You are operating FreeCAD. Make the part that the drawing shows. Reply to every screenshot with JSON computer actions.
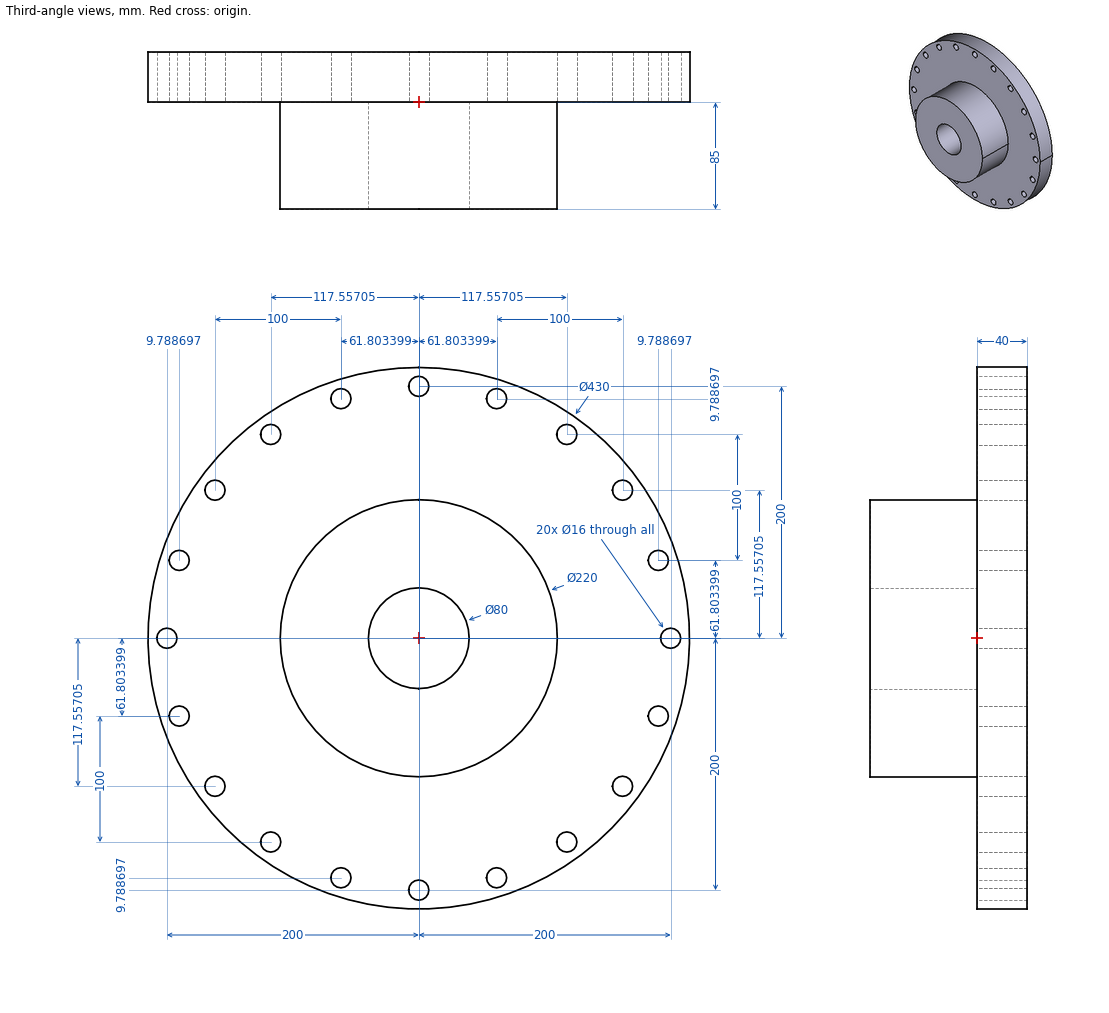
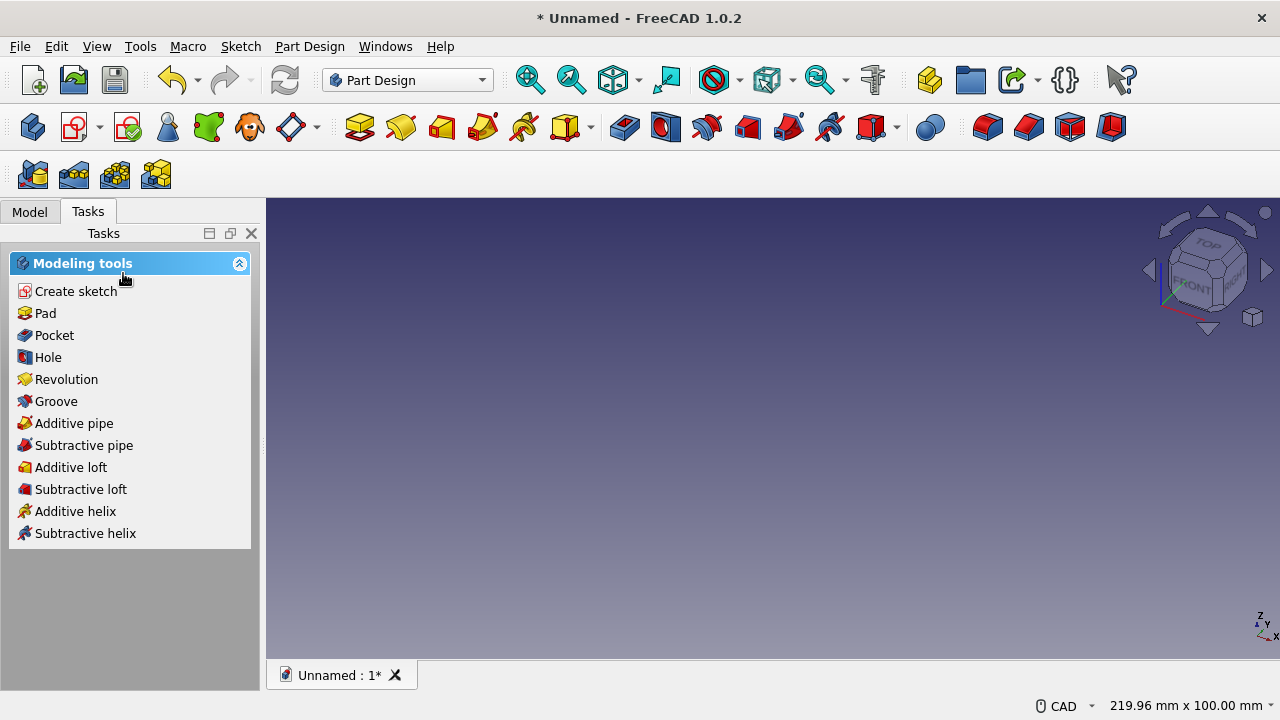
{"action": "left_click", "coordinate": [360, 128]}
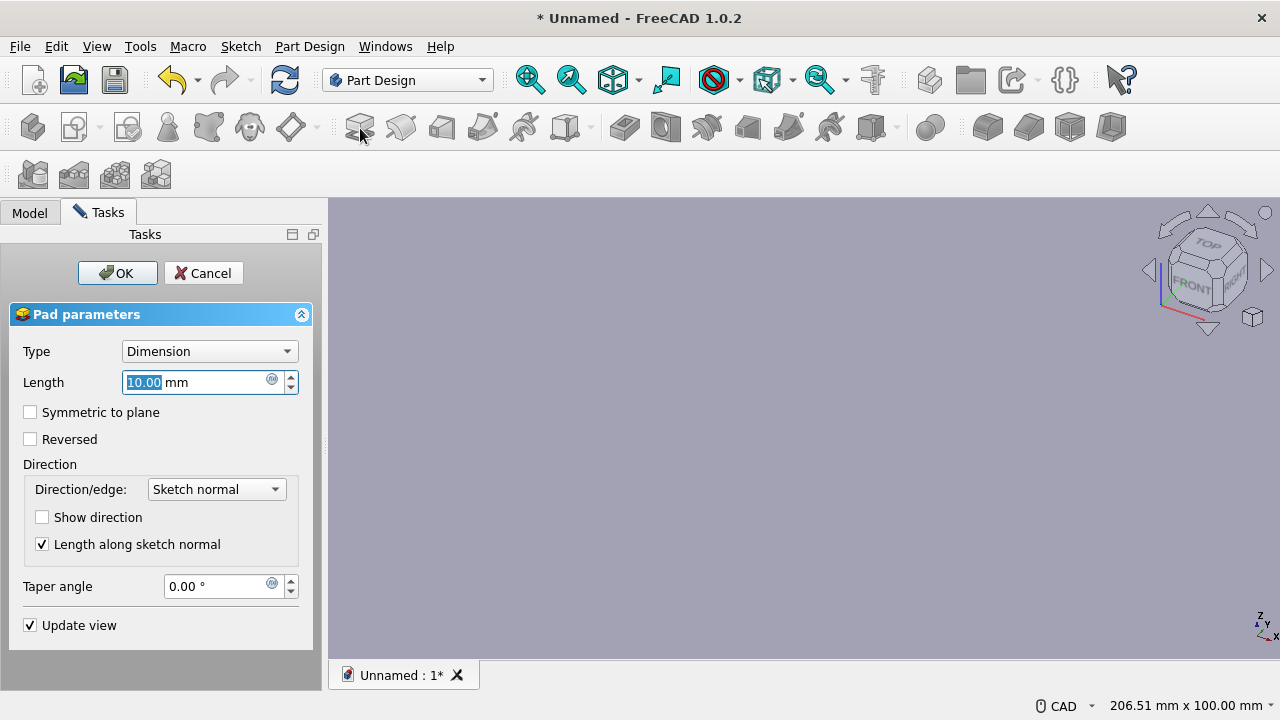
{"action": "type", "text": "40"}
{"action": "key", "text": "Tab"}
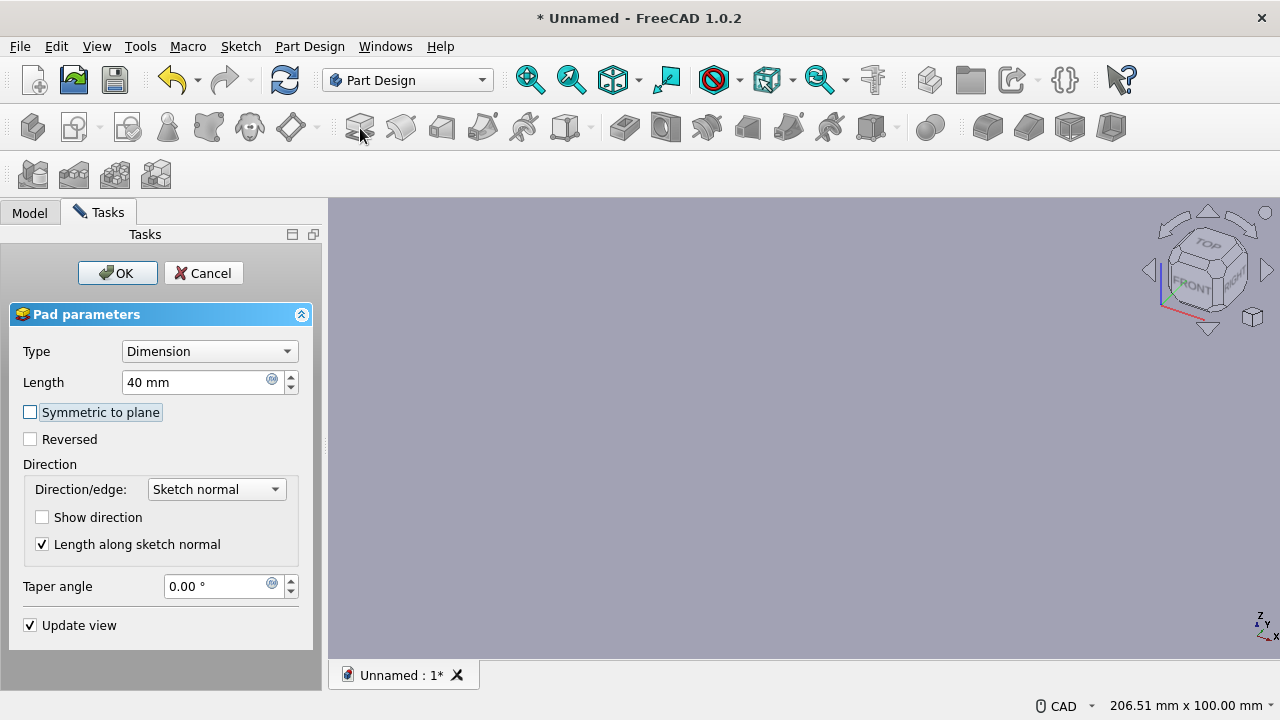
{"action": "left_click", "coordinate": [31, 439]}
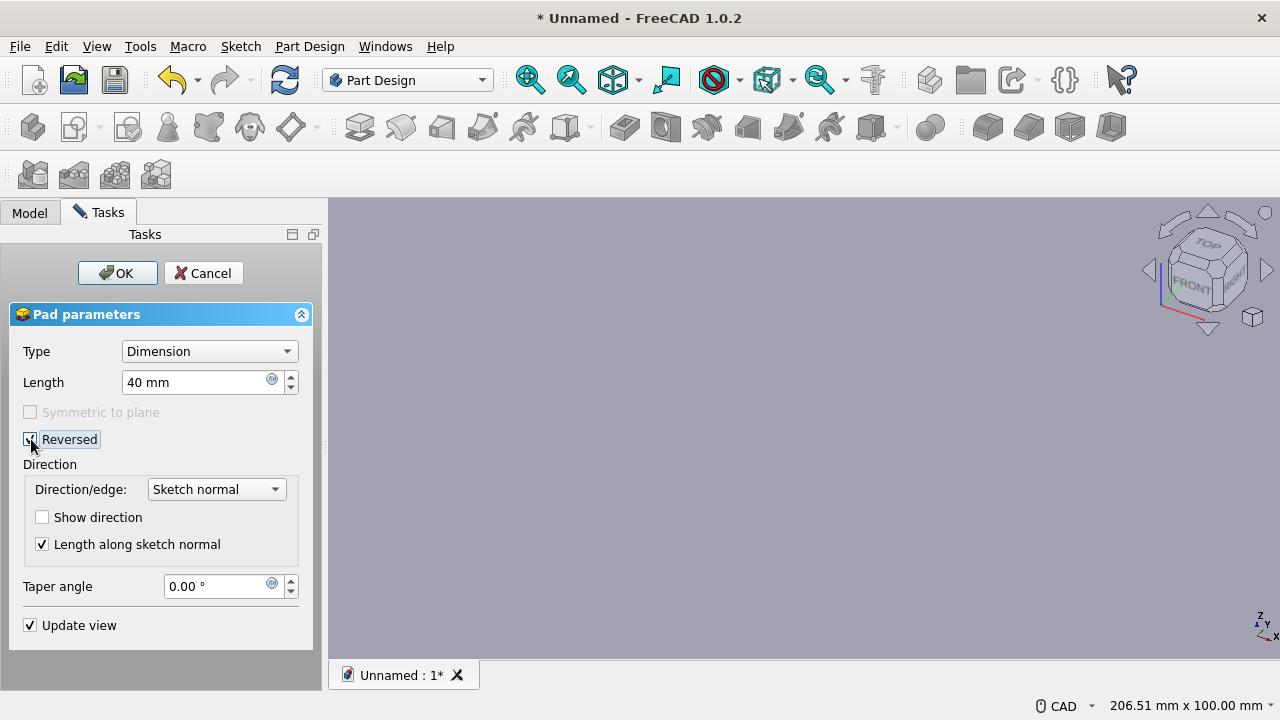
{"action": "left_click", "coordinate": [118, 273]}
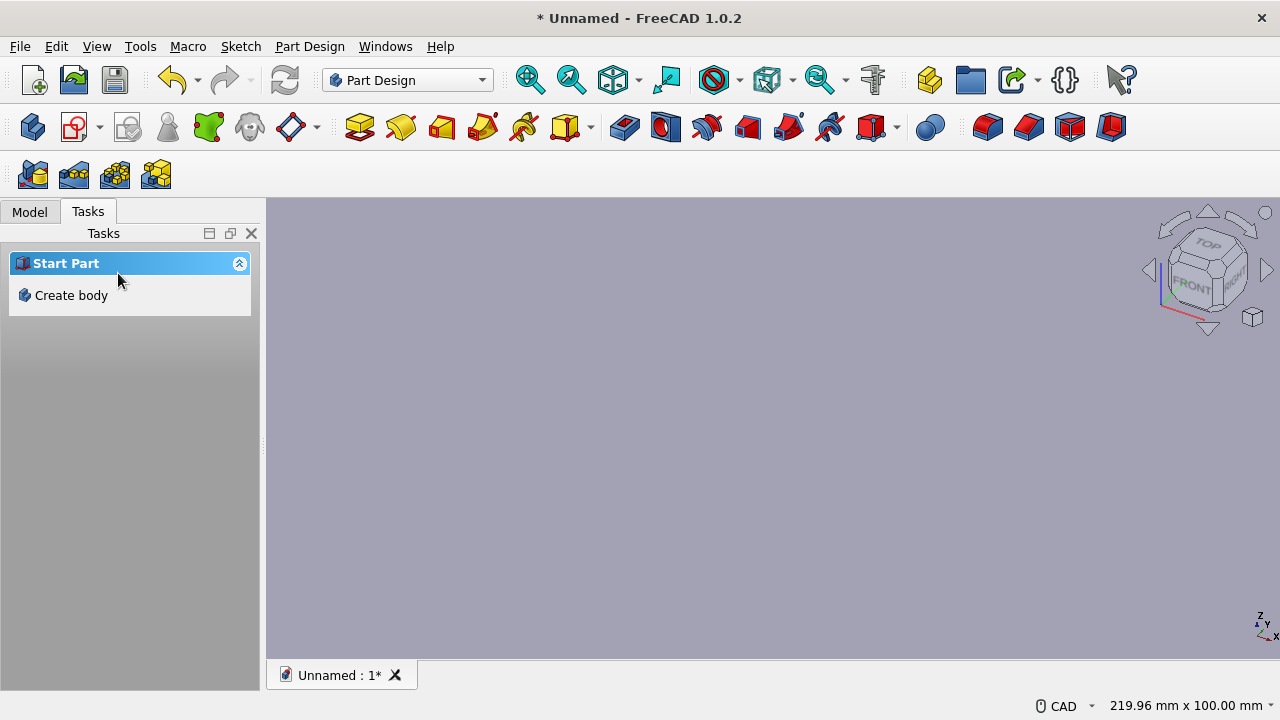
{"action": "left_click", "coordinate": [531, 80]}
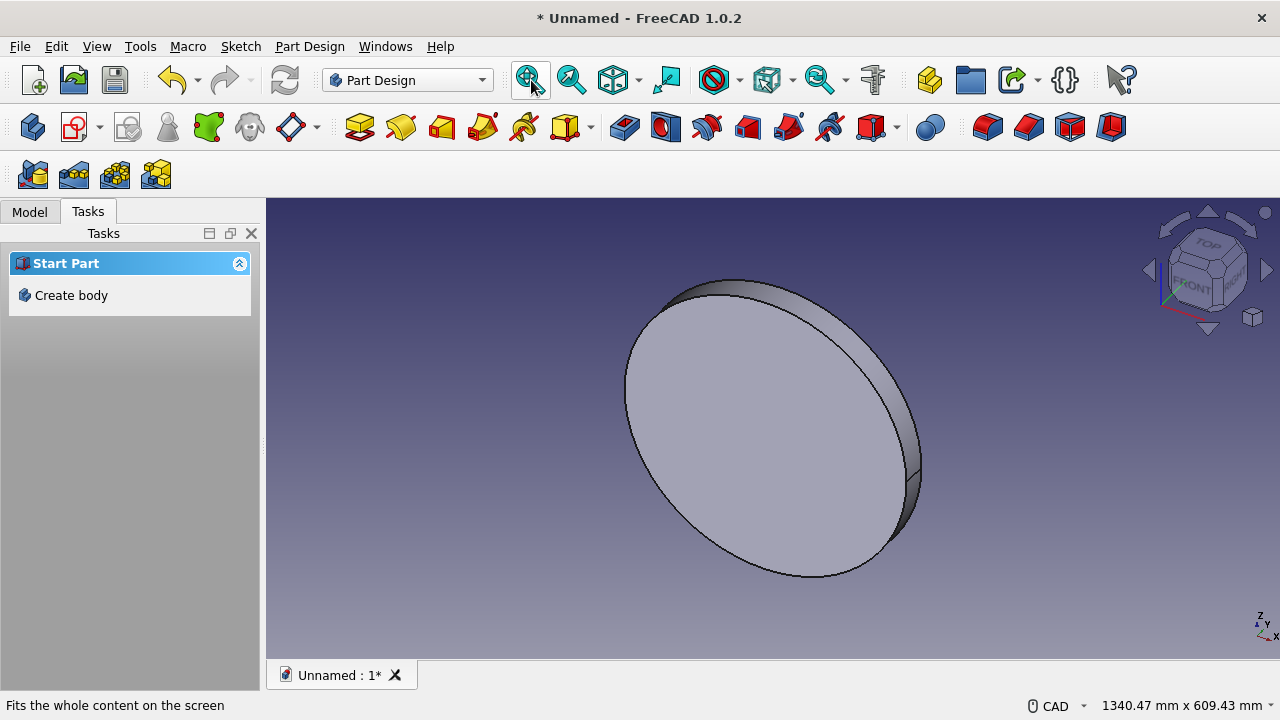
{"action": "key", "text": "4"}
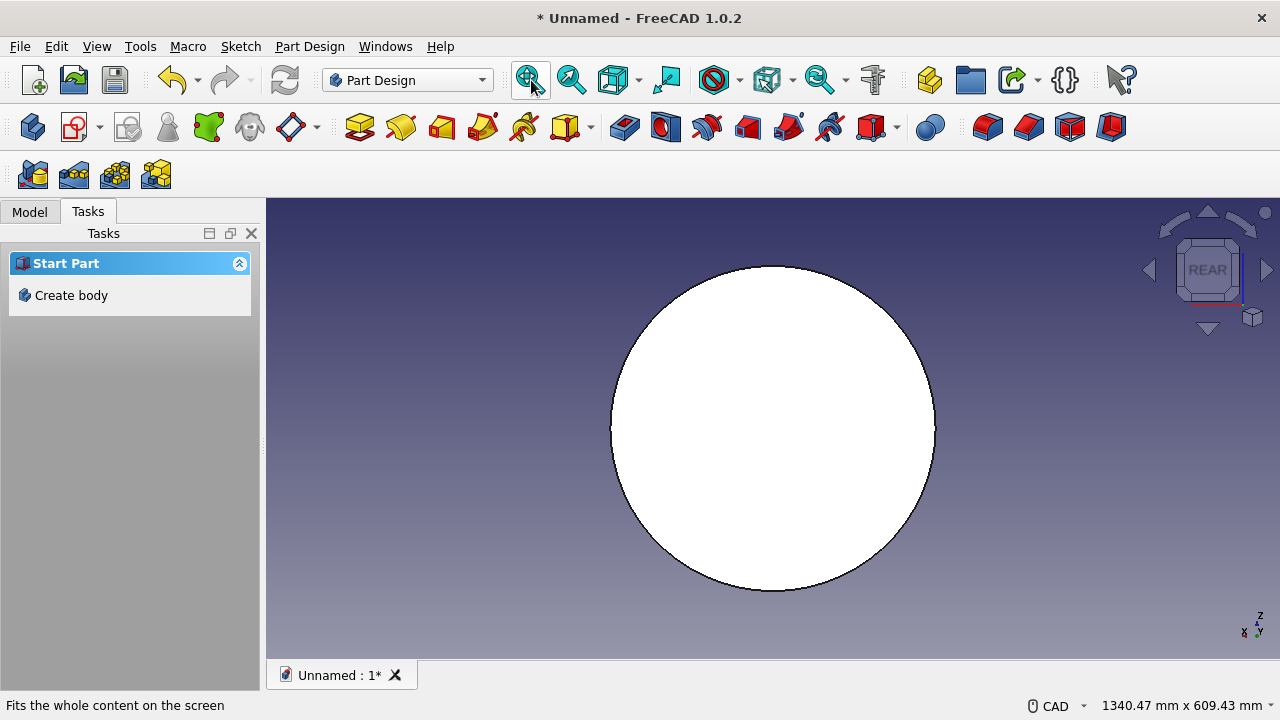
{"action": "left_click", "coordinate": [773, 428]}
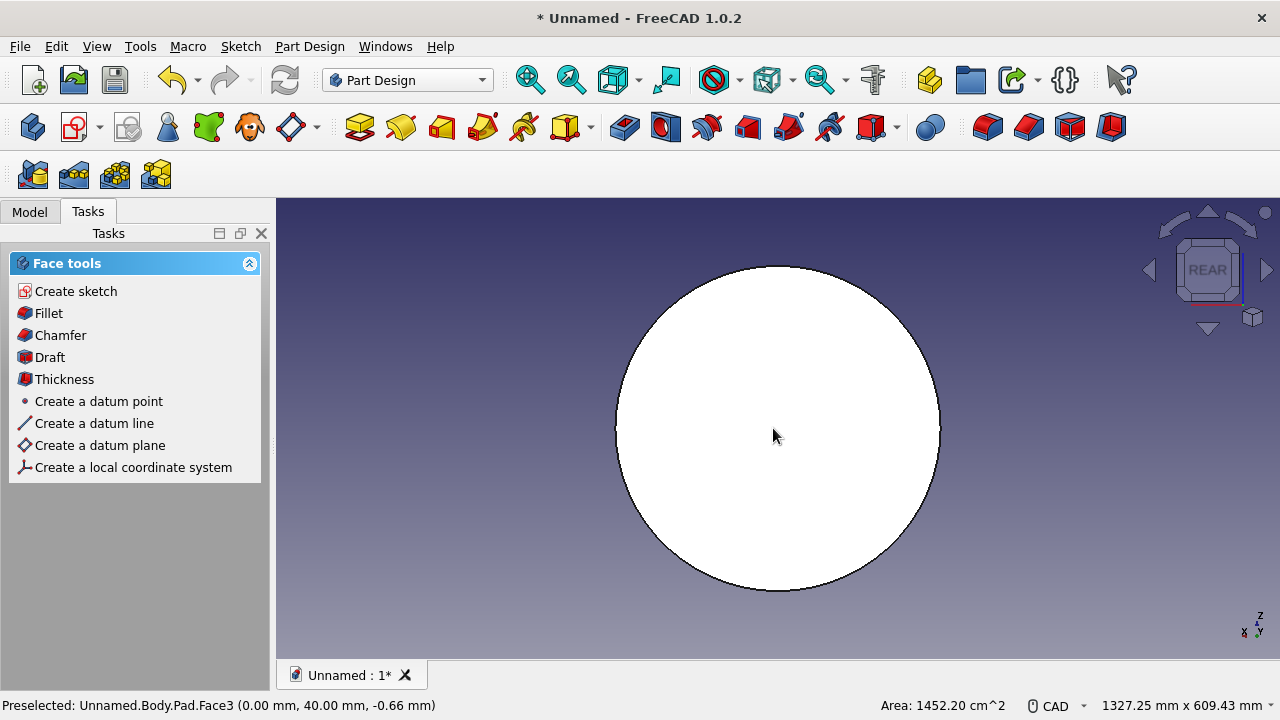
{"action": "left_click", "coordinate": [74, 128]}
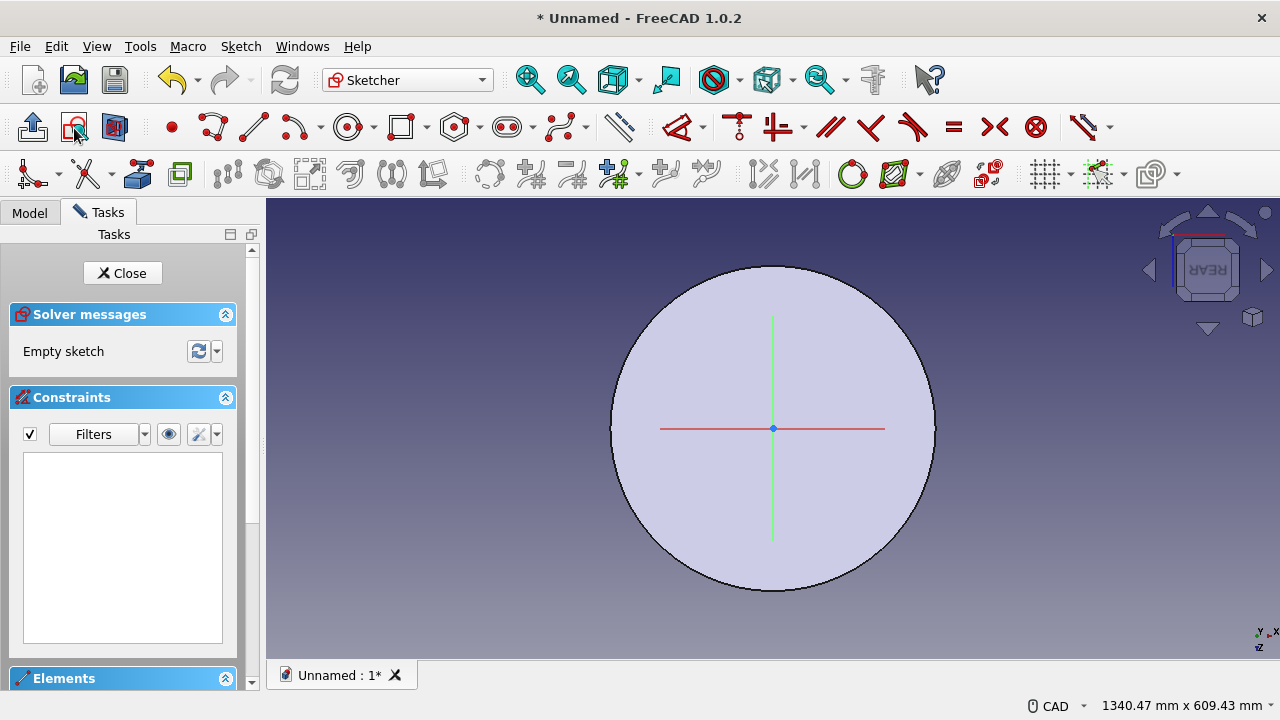
{"action": "left_click", "coordinate": [348, 128]}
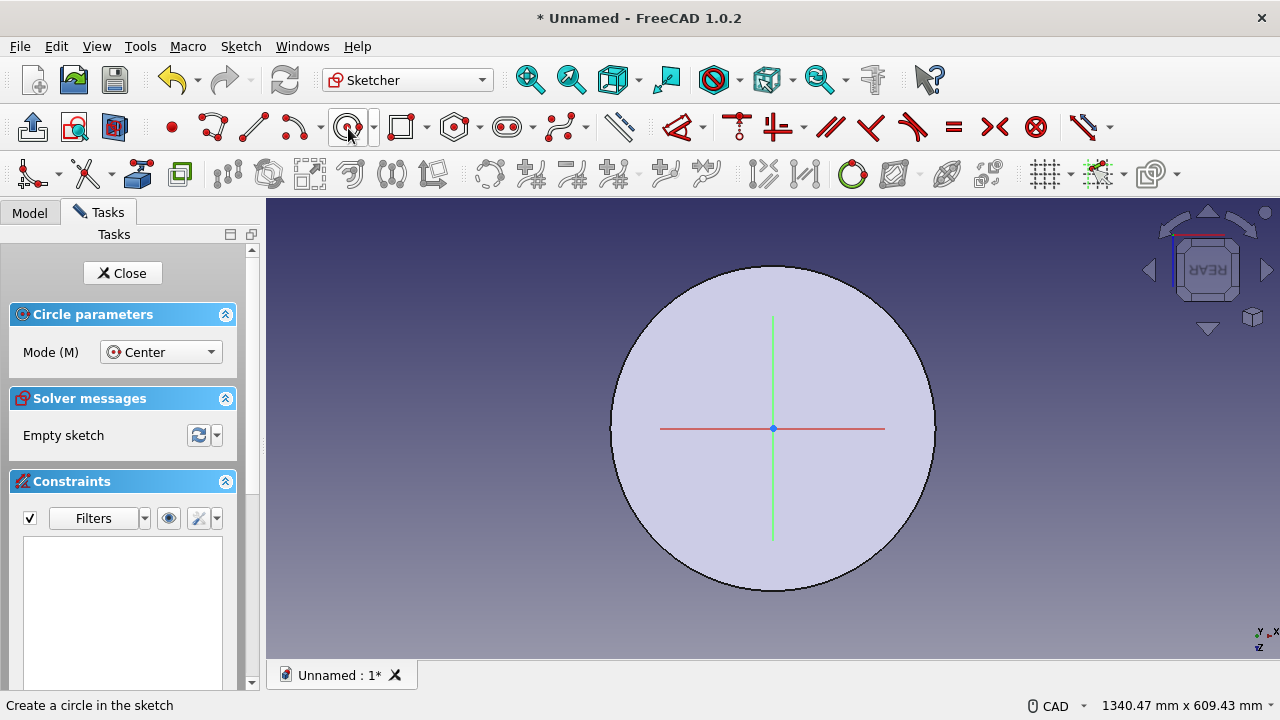
{"action": "scroll", "coordinate": [924, 428], "scroll_direction": "up", "scroll_amount": 7}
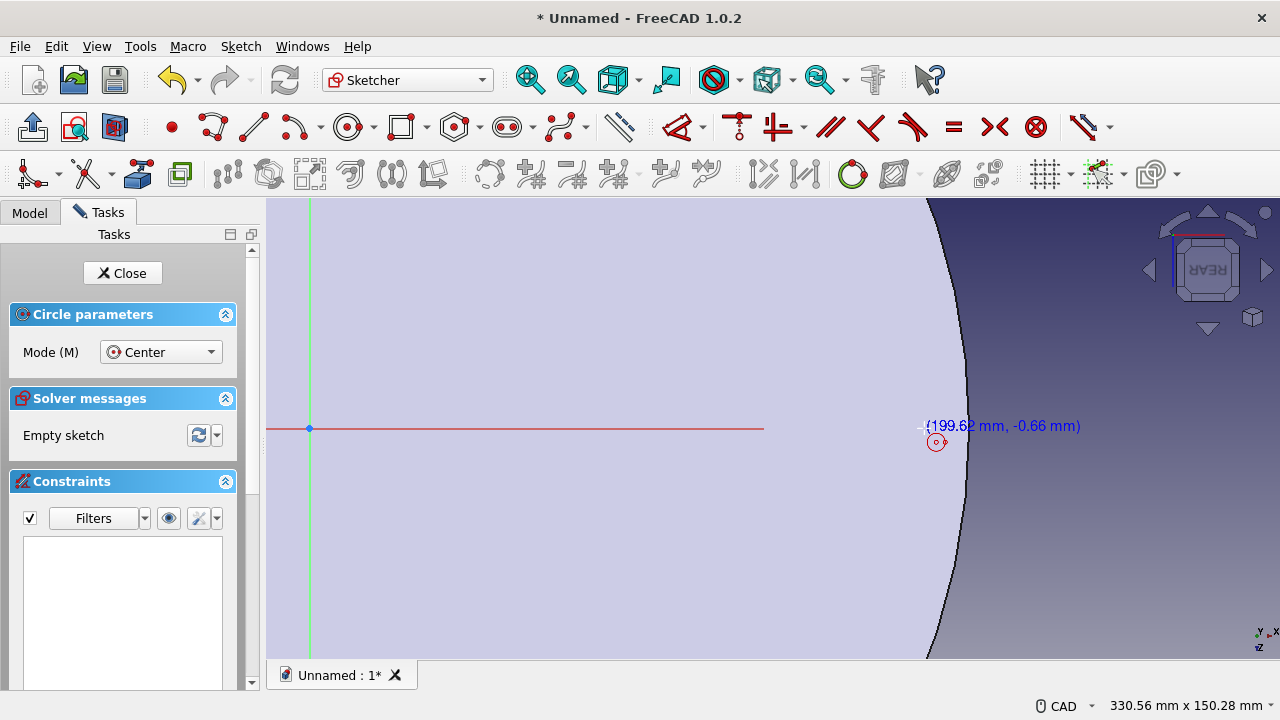
{"action": "scroll", "coordinate": [834, 429], "scroll_direction": "down", "scroll_amount": 7}